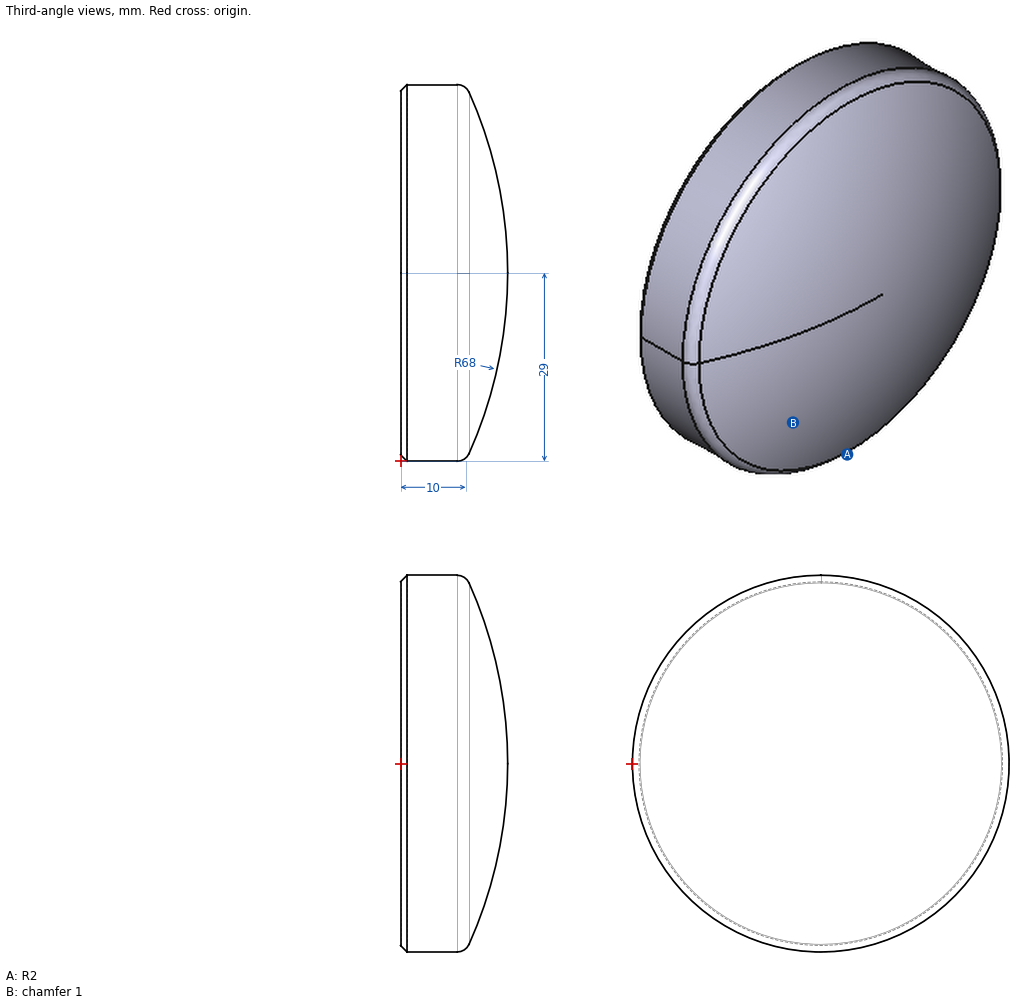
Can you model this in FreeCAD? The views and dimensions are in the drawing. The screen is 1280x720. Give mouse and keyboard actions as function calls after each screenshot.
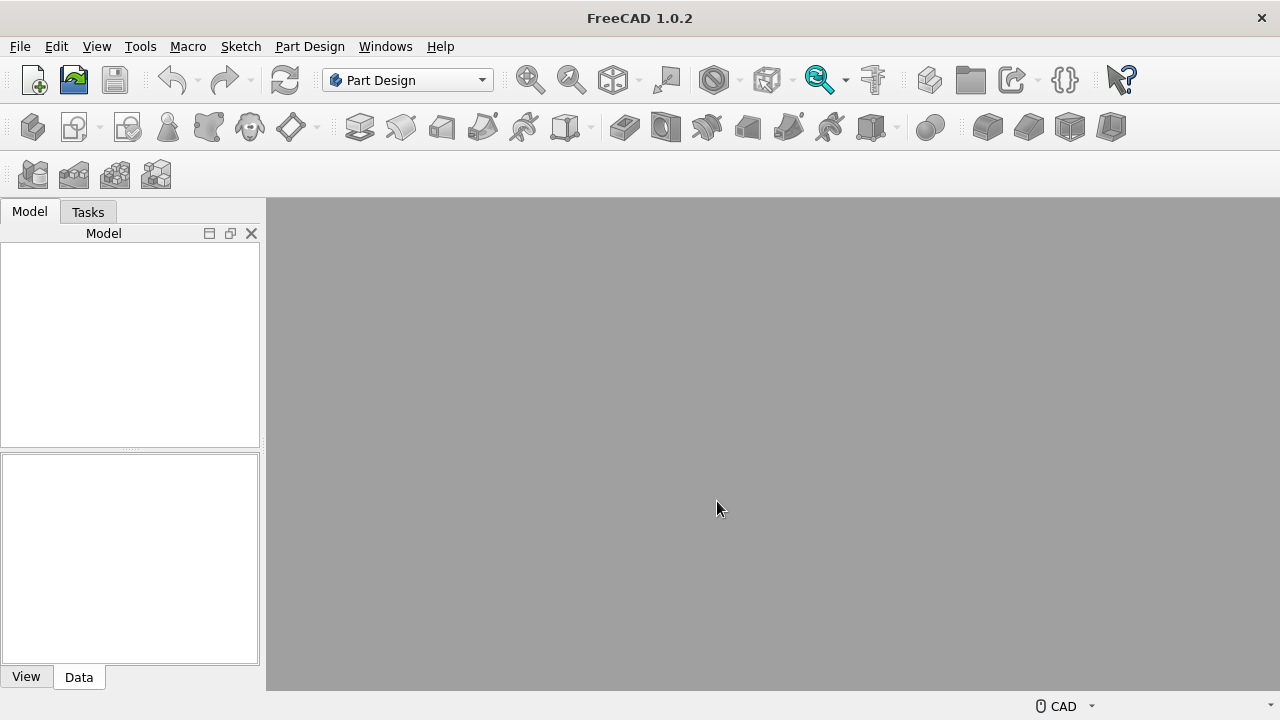
click(33, 80)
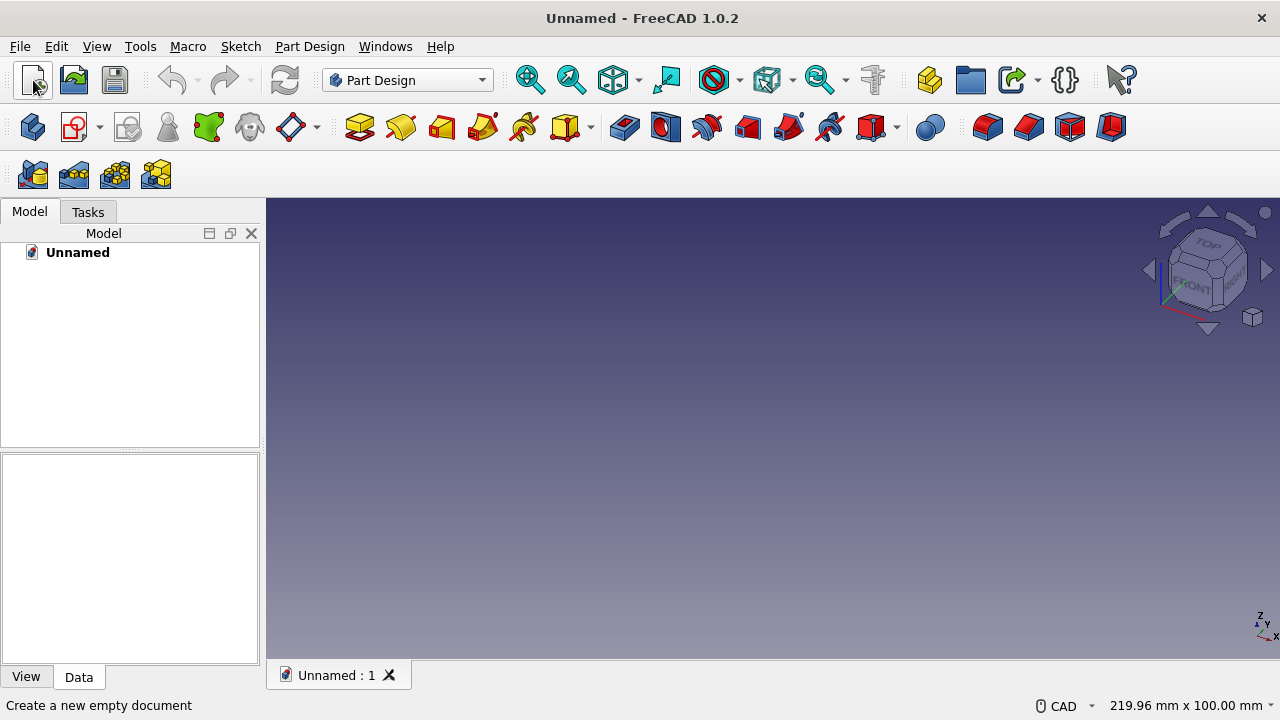
click(74, 128)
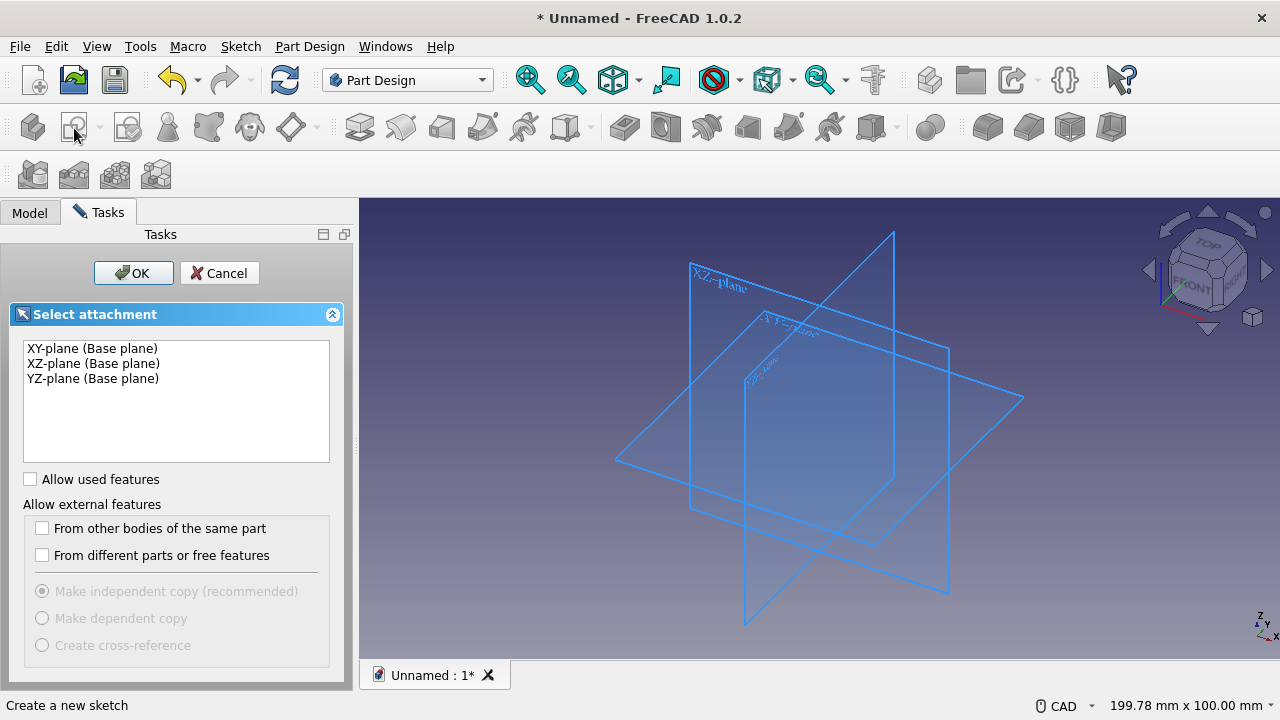
click(84, 348)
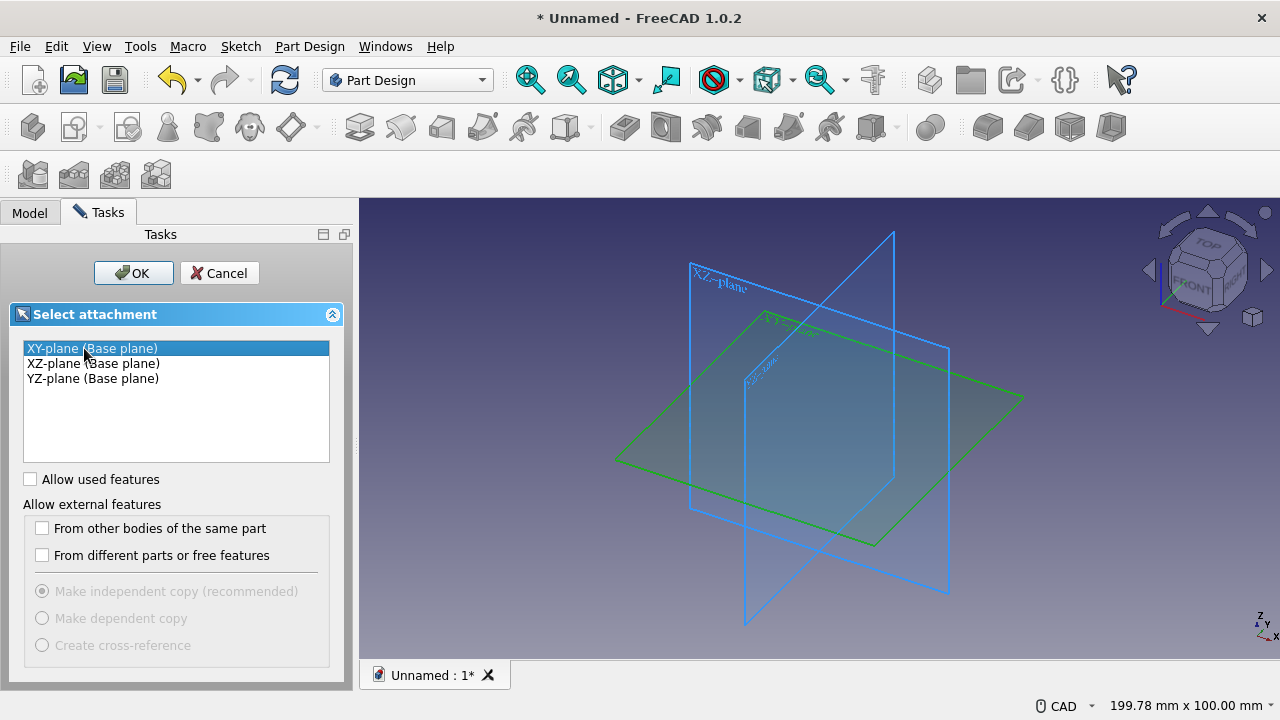
click(134, 273)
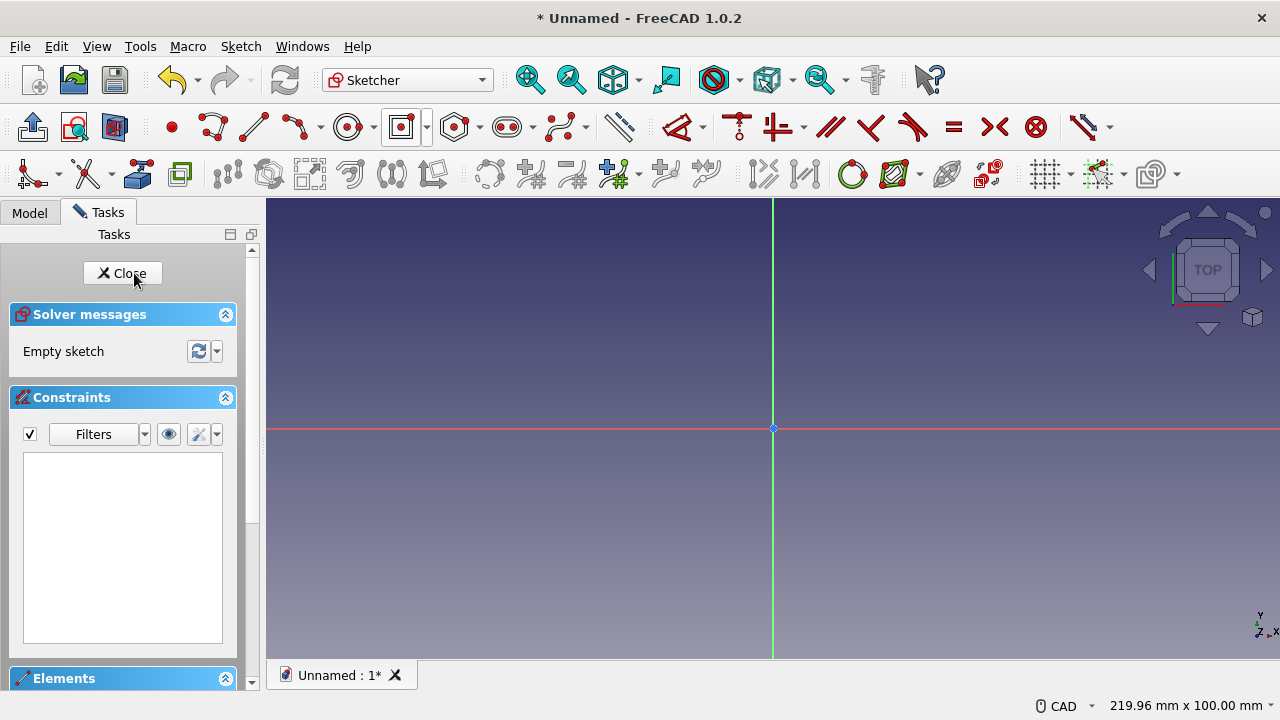
scroll(926, 307, up, 4)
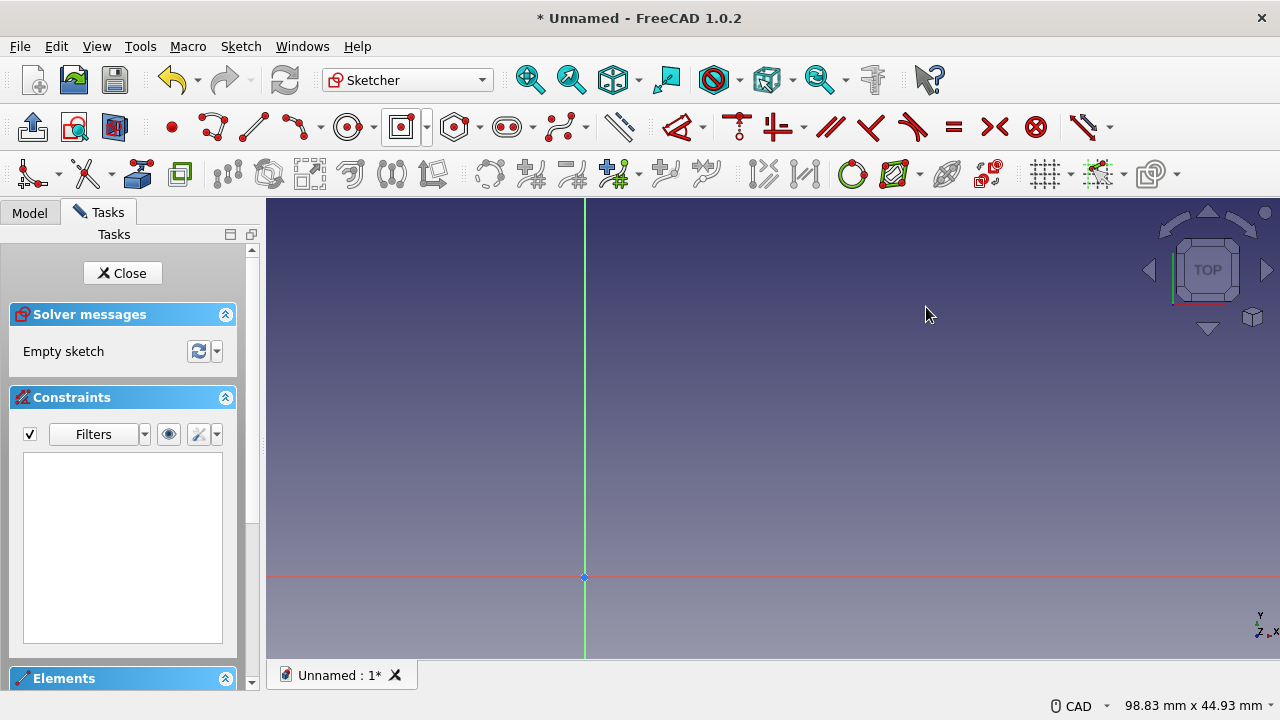
click(213, 128)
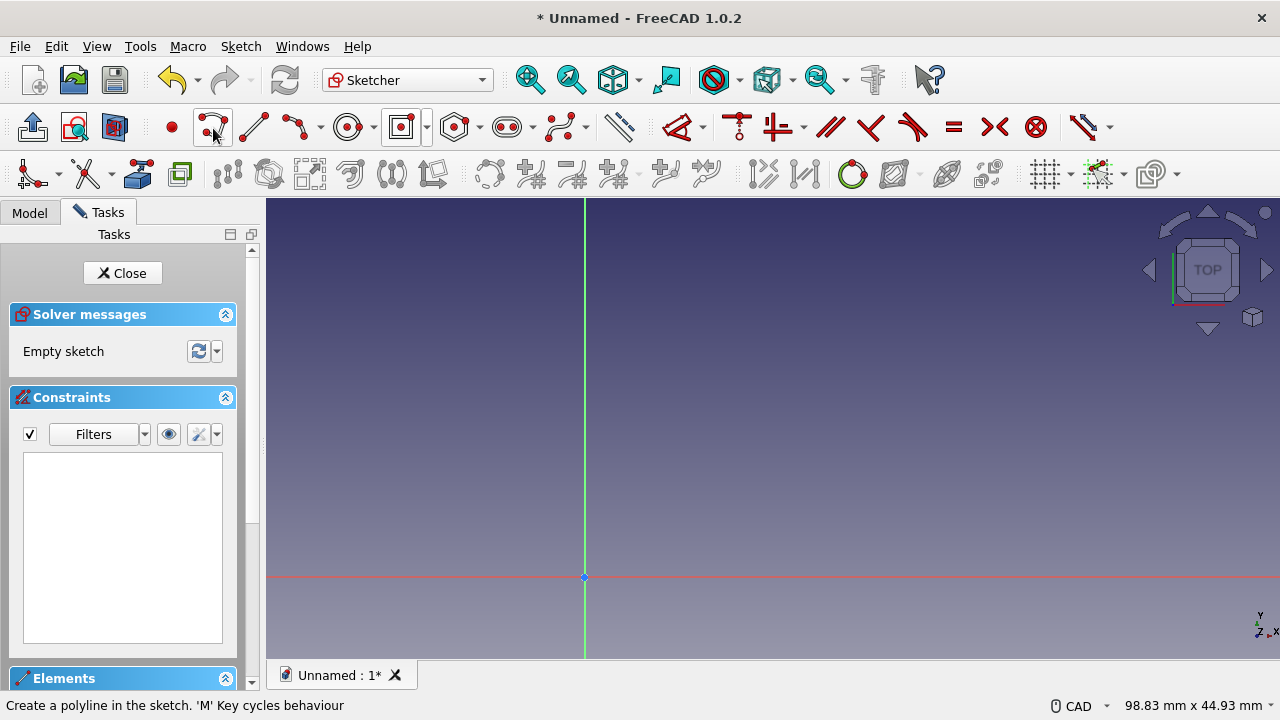
click(754, 280)
click(585, 280)
click(585, 577)
click(687, 568)
right_click(687, 568)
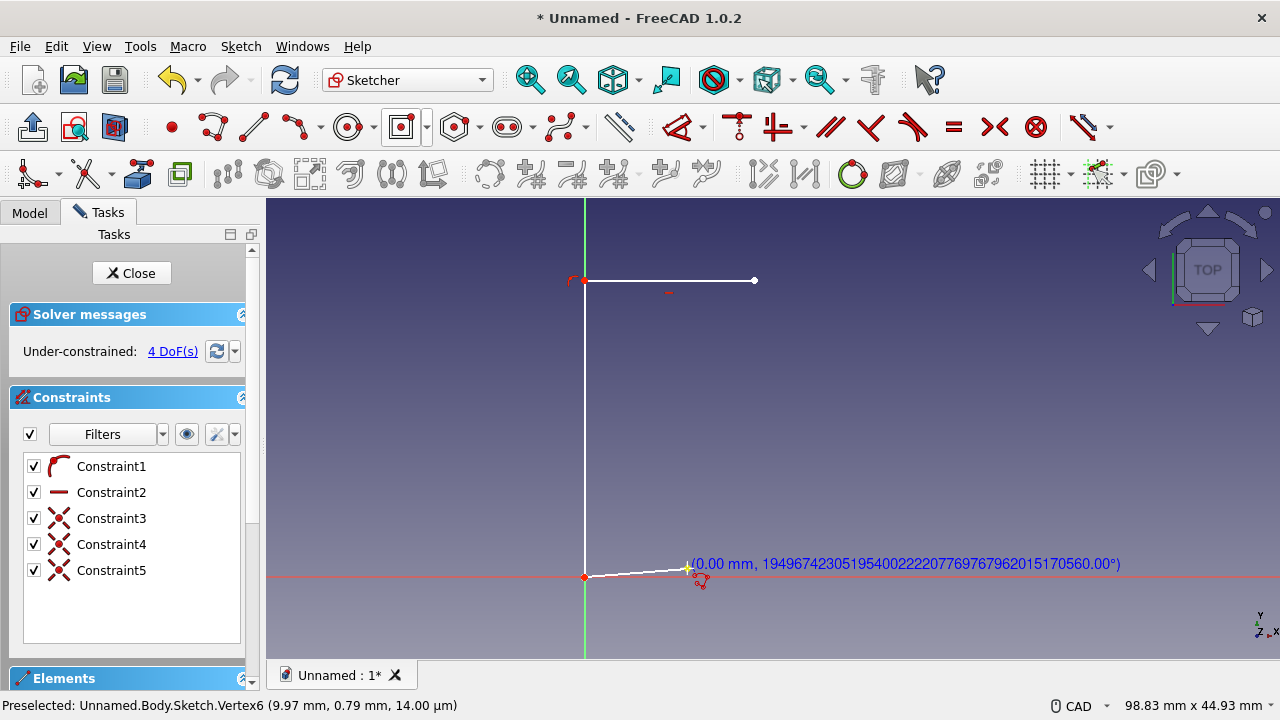
click(294, 128)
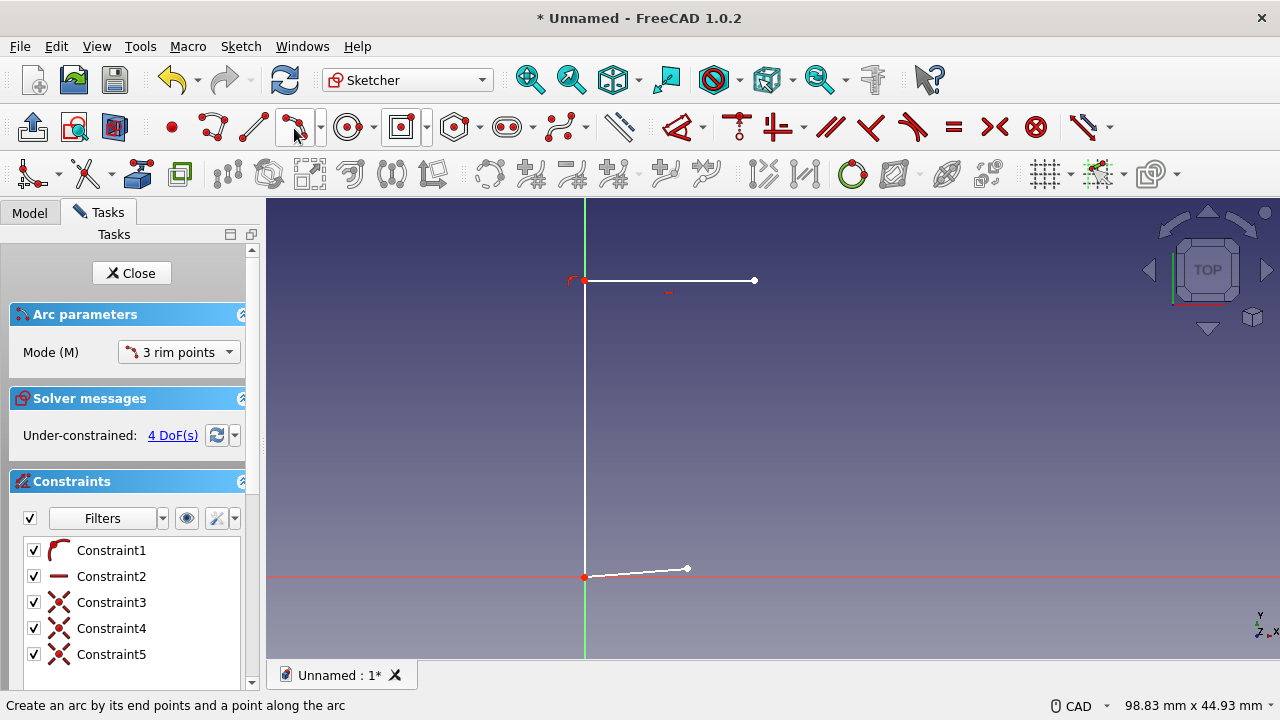
click(687, 569)
click(754, 281)
click(737, 432)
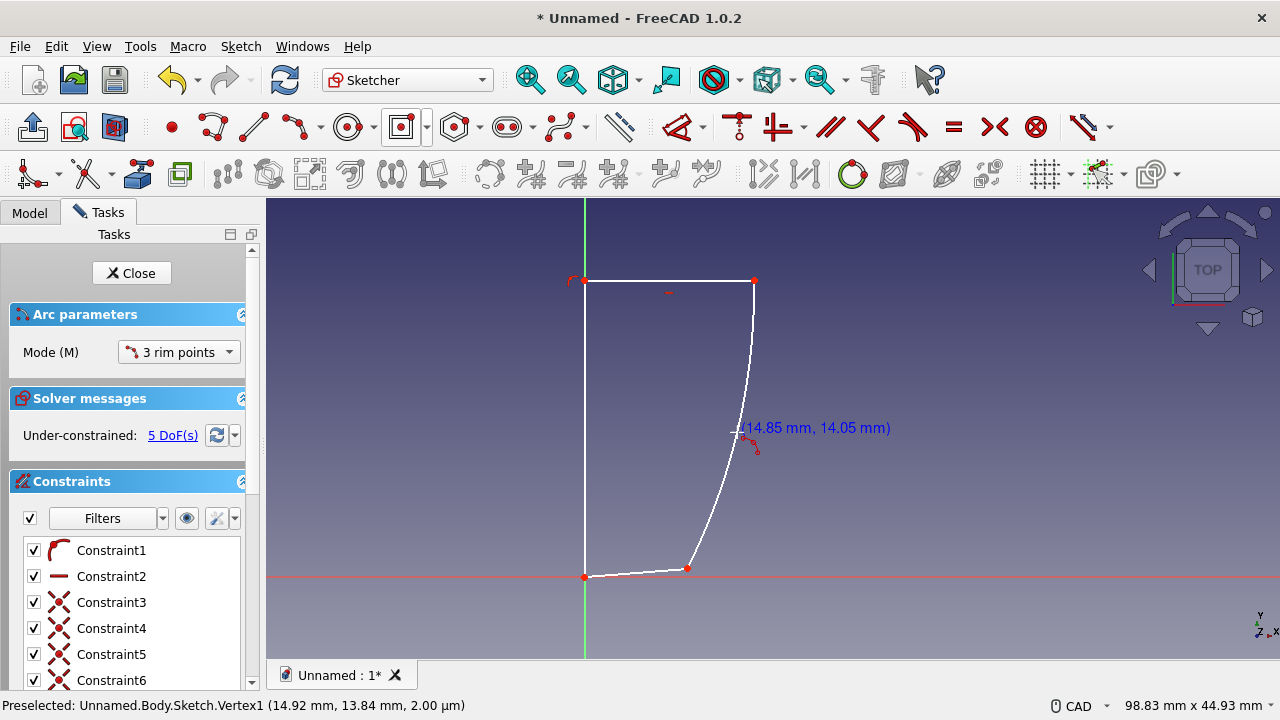
click(254, 128)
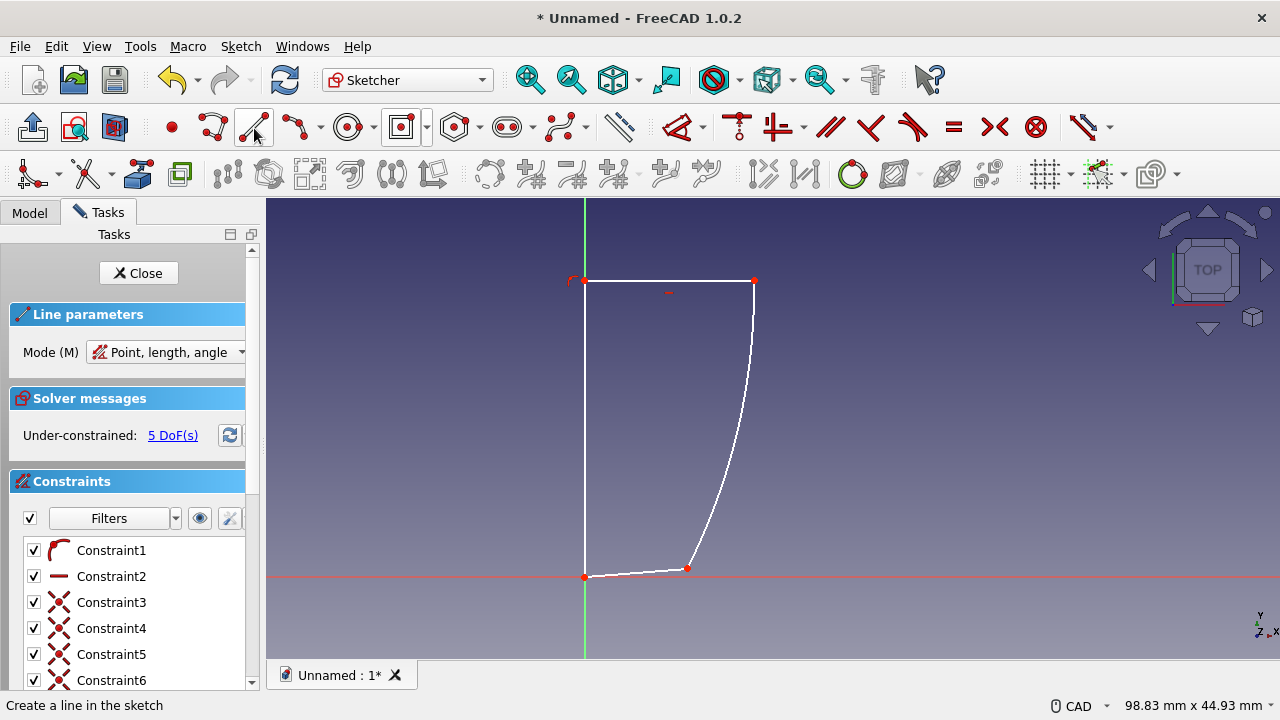
click(771, 280)
click(822, 280)
key(Escape)